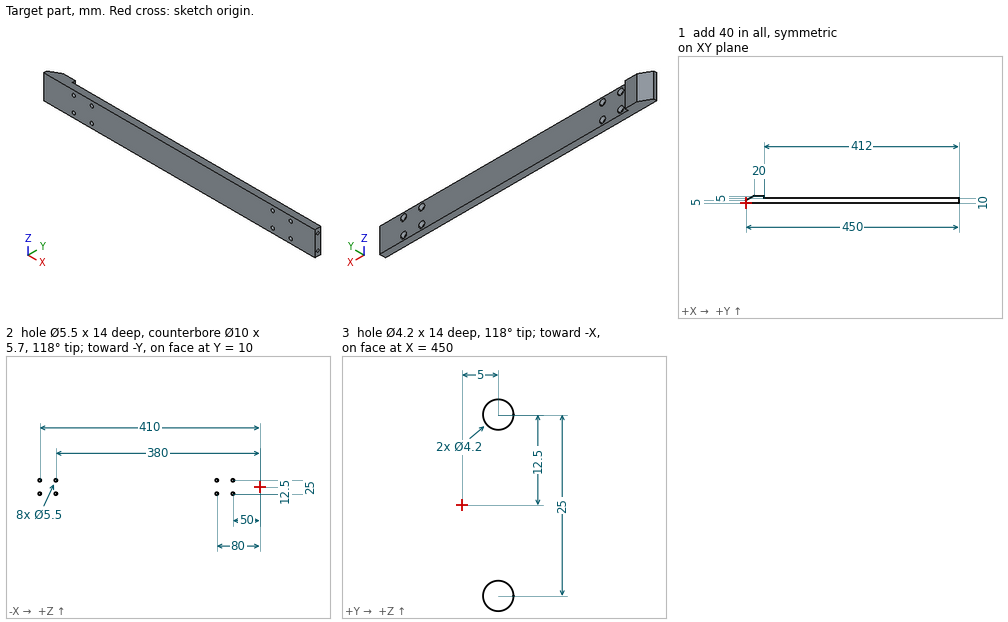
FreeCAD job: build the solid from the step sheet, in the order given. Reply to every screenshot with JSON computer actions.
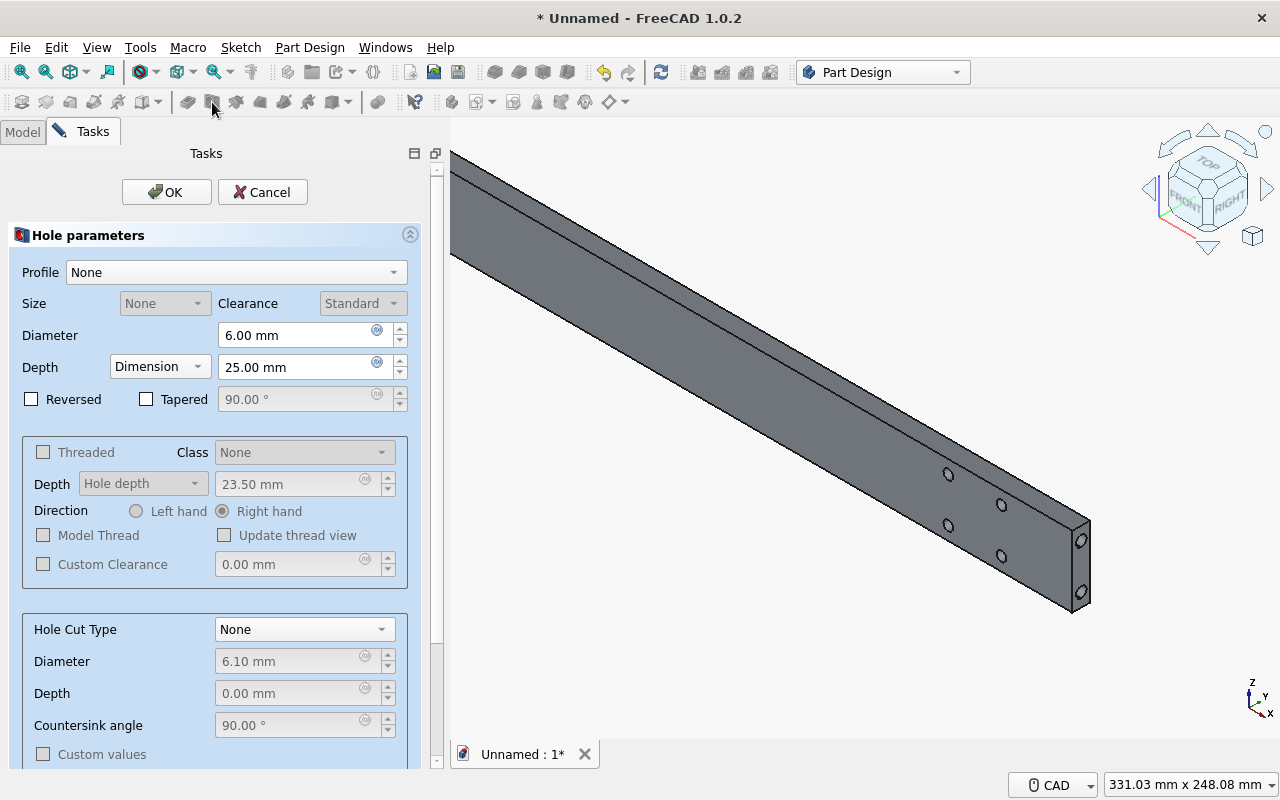
{"action": "triple_click", "coordinate": [305, 335]}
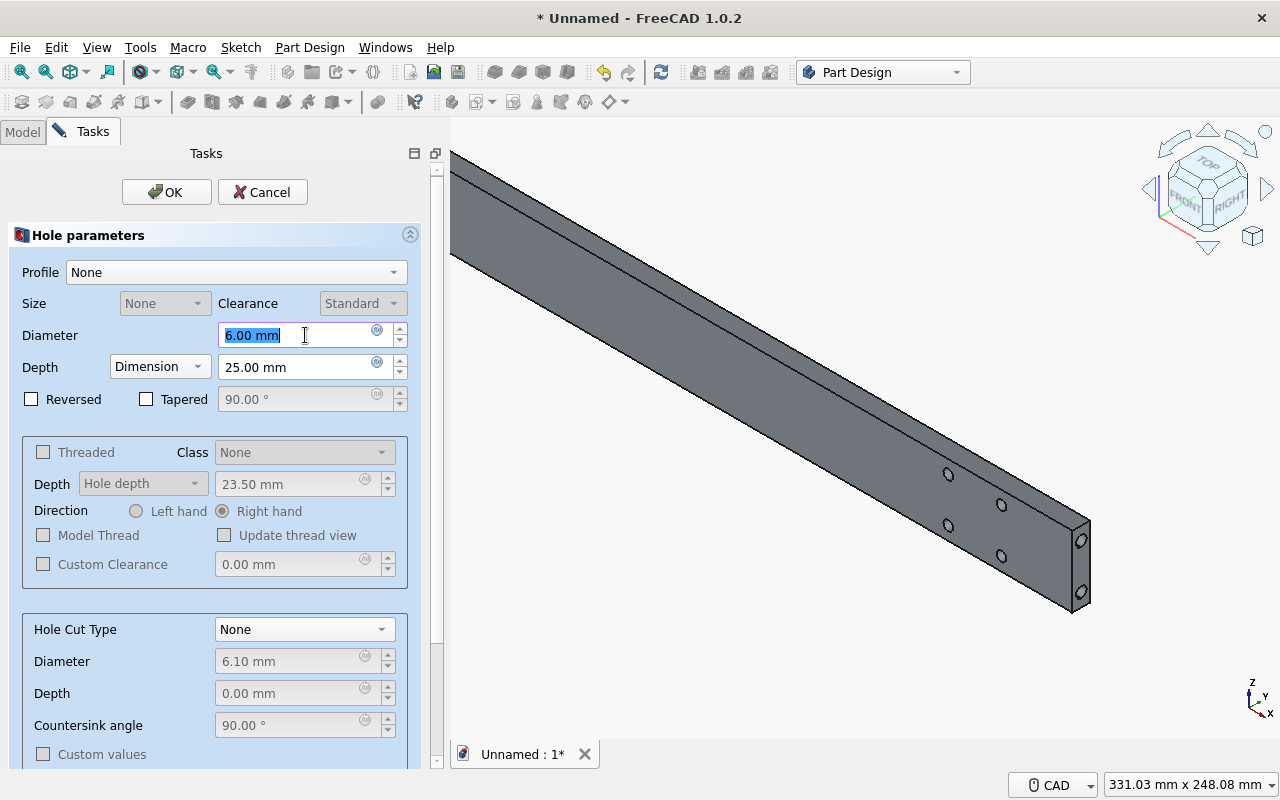
{"action": "type", "text": "4.2"}
{"action": "key", "text": "Tab"}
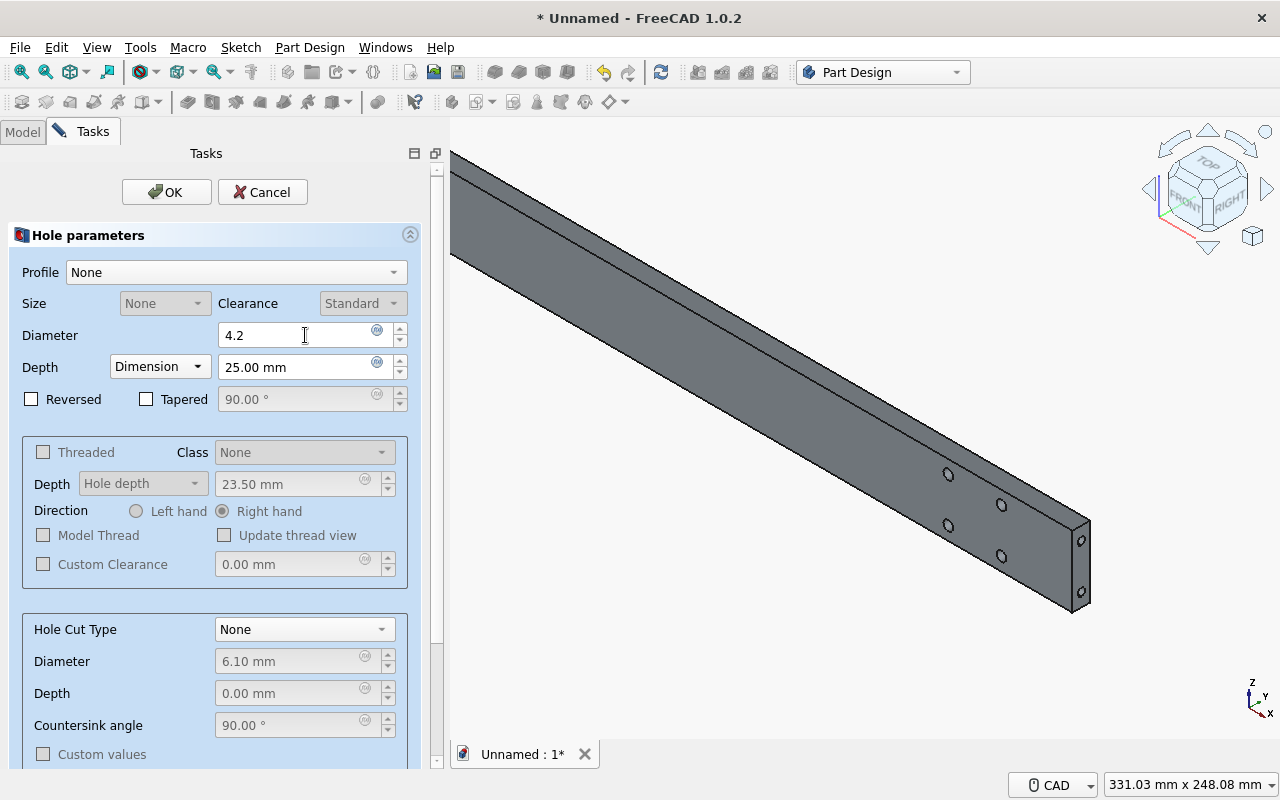
{"action": "triple_click", "coordinate": [305, 367]}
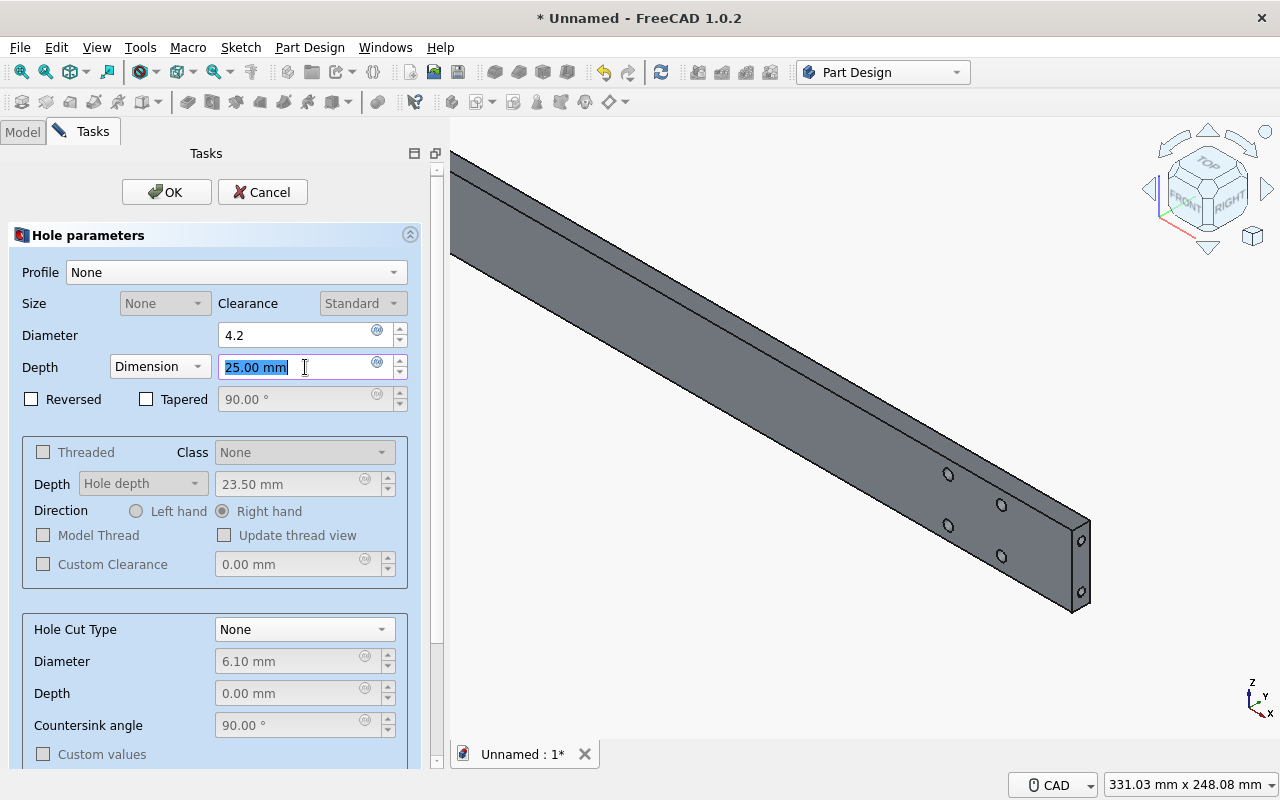
{"action": "type", "text": "14"}
{"action": "key", "text": "Tab"}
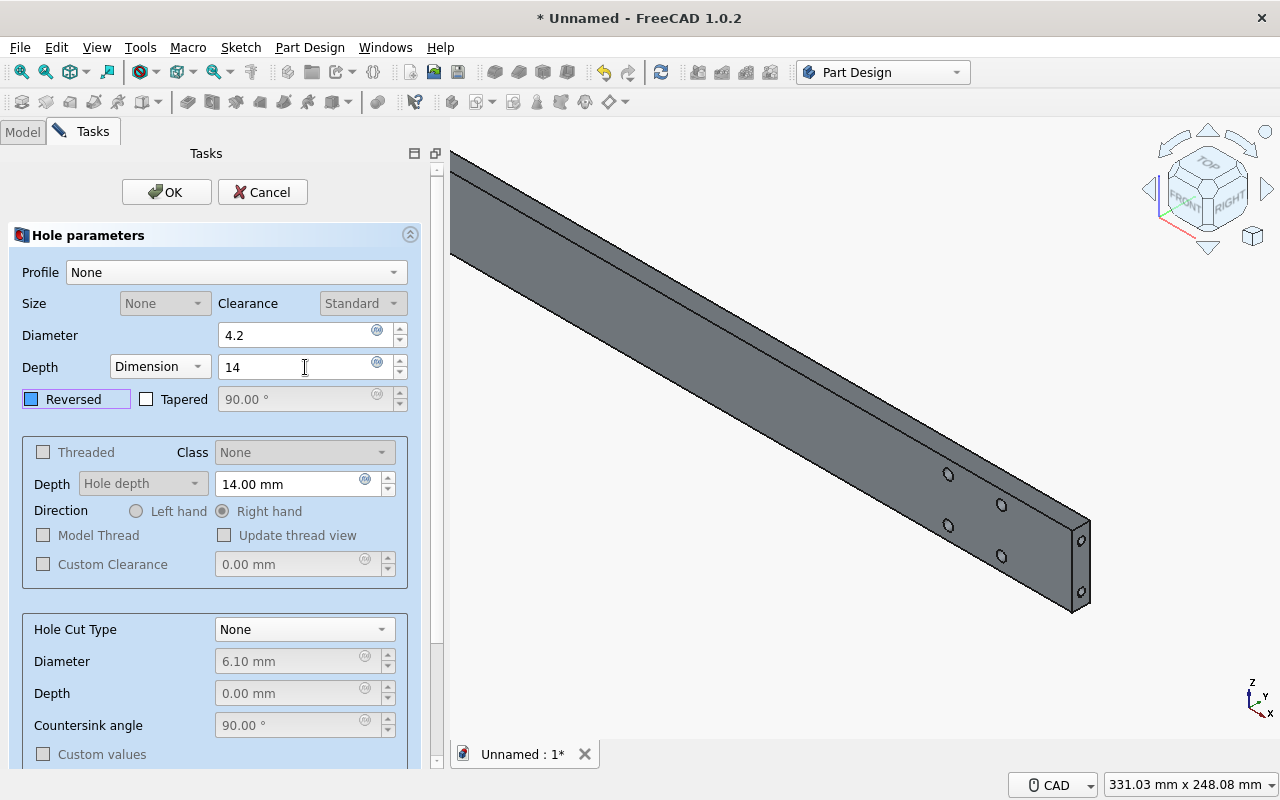
{"action": "left_click", "coordinate": [167, 192]}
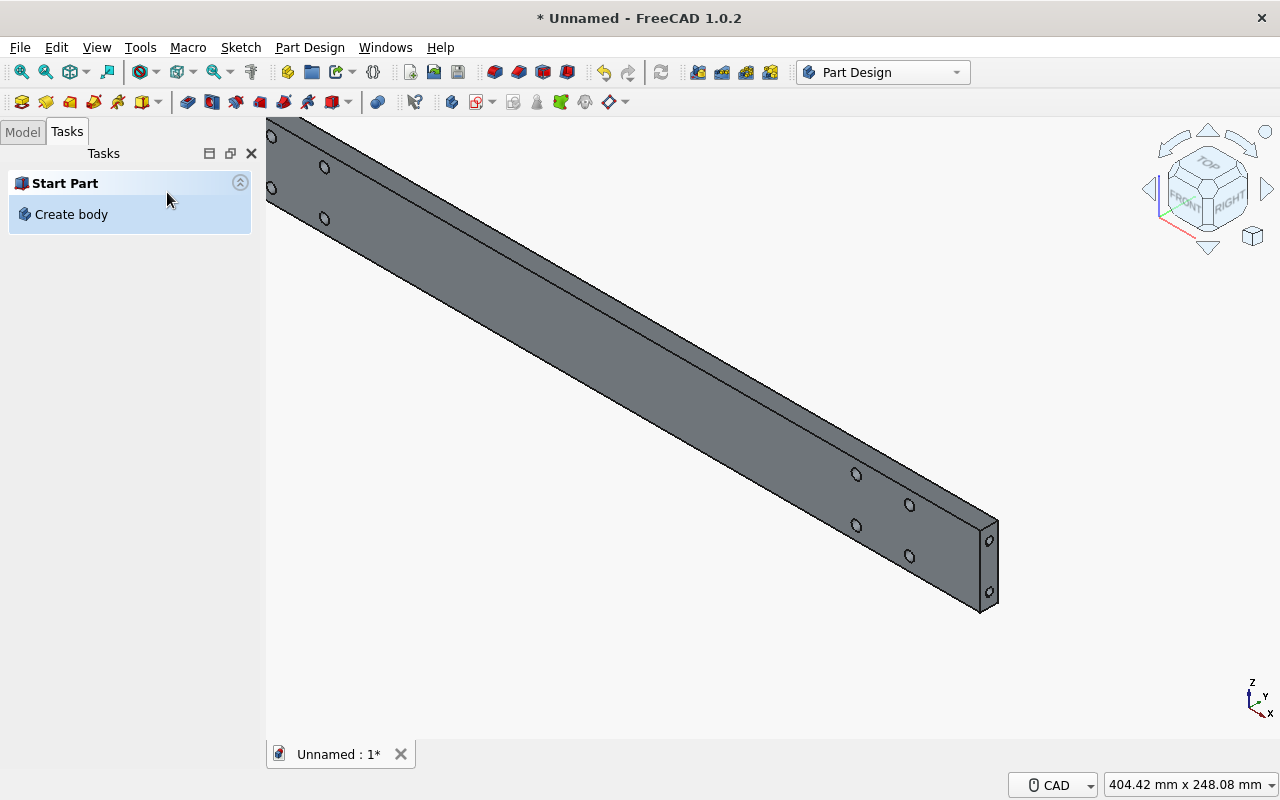
{"action": "left_click", "coordinate": [22, 72]}